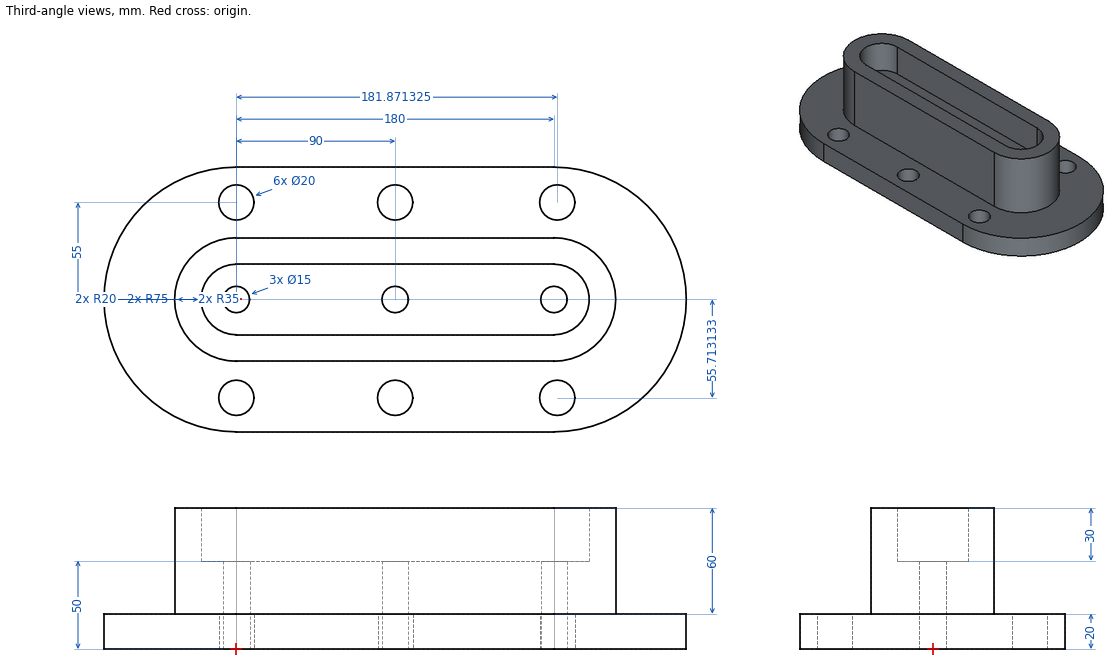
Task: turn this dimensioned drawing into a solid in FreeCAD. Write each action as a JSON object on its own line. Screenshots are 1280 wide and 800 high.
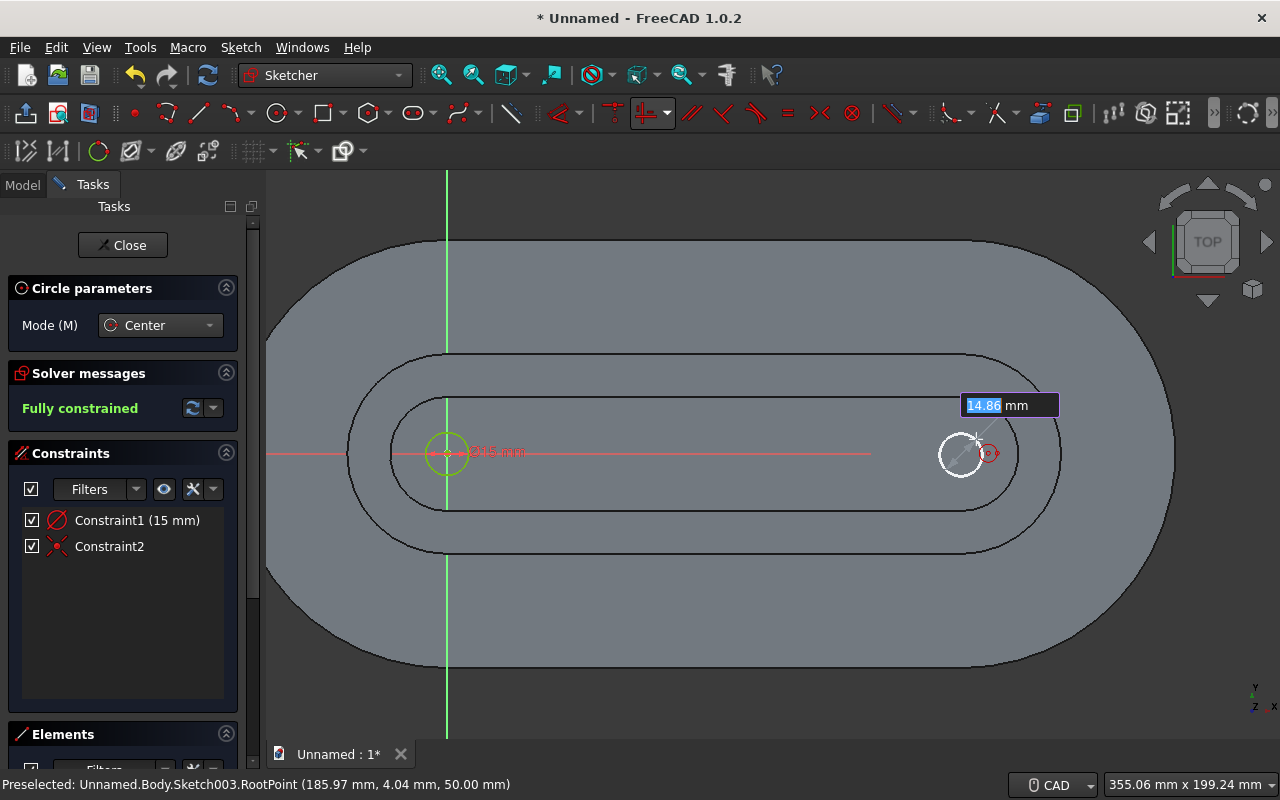
{"action": "type", "text": "15"}
{"action": "key", "text": "Return"}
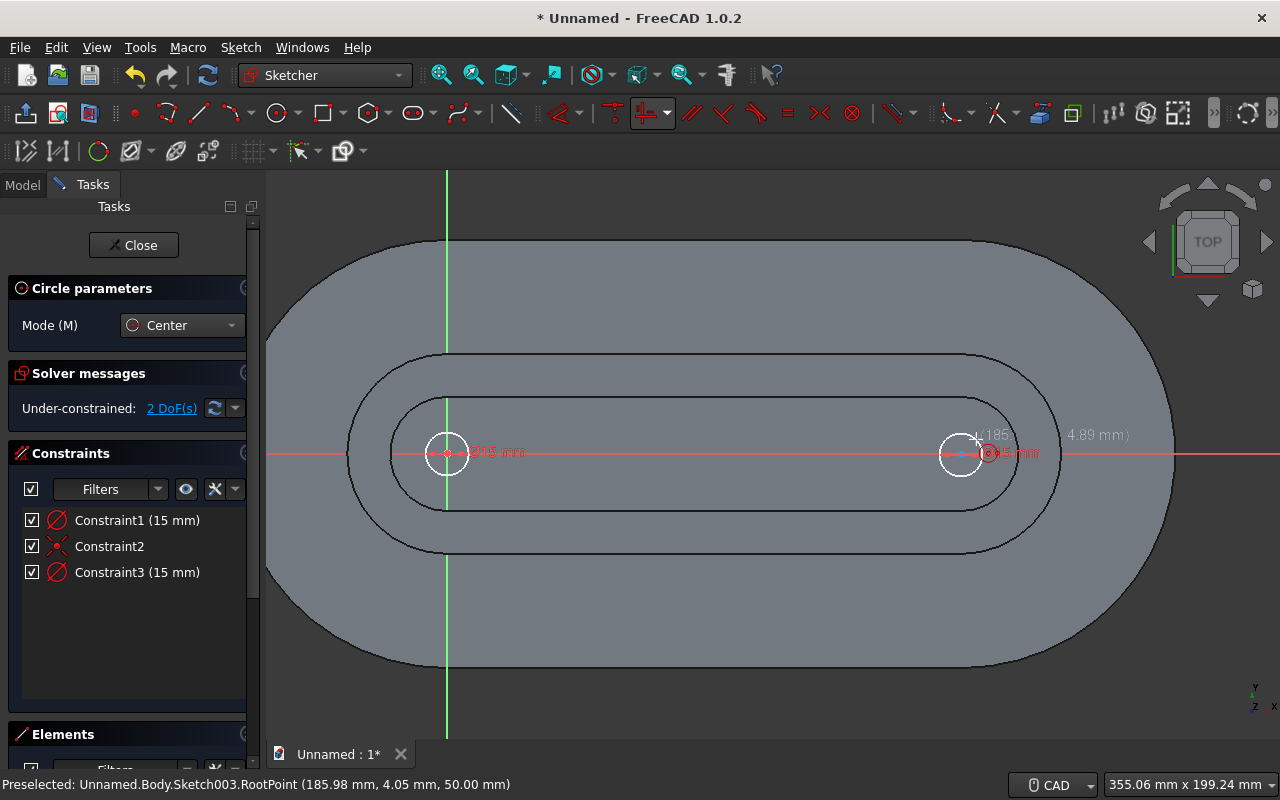
{"action": "left_click", "coordinate": [704, 454]}
{"action": "mouse_move", "coordinate": [719, 439]}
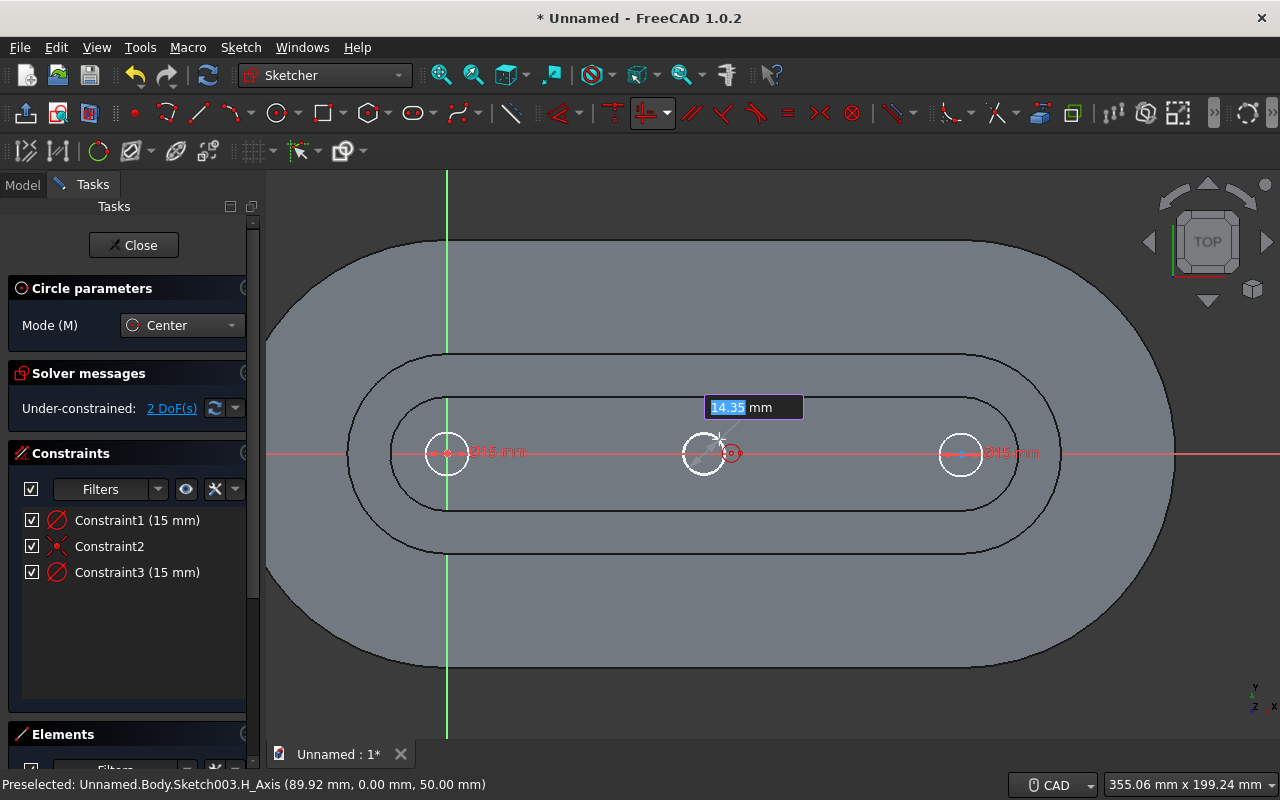
{"action": "type", "text": "15"}
{"action": "key", "text": "Return"}
{"action": "key", "text": "Escape"}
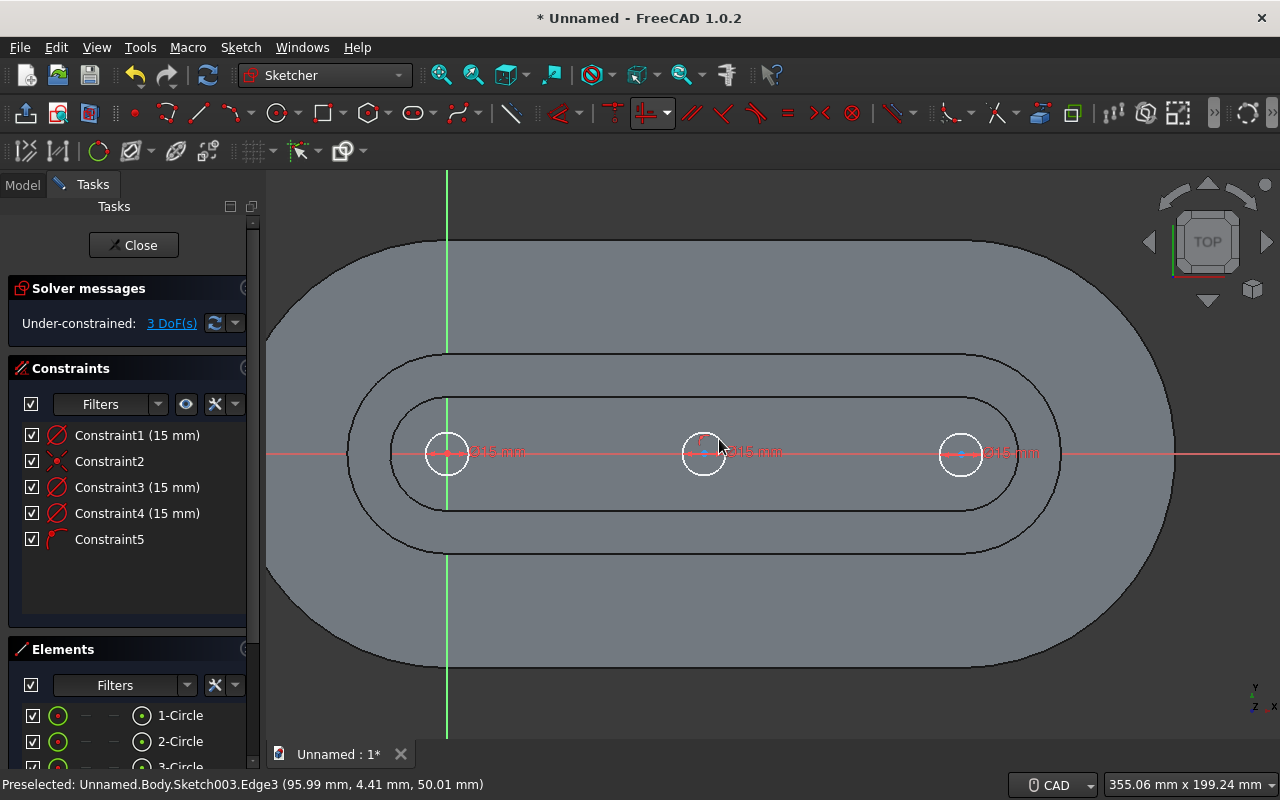
{"action": "left_click", "coordinate": [961, 455]}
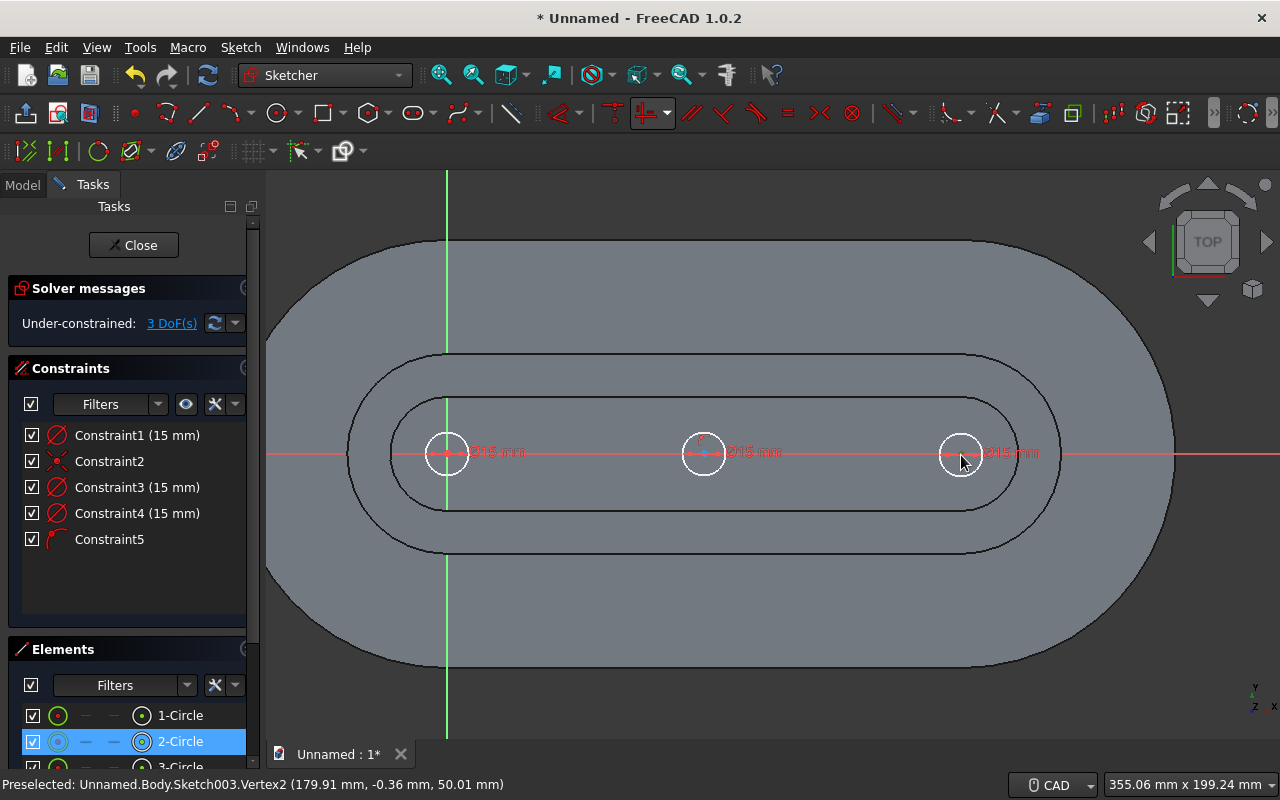
{"action": "left_click", "coordinate": [353, 454]}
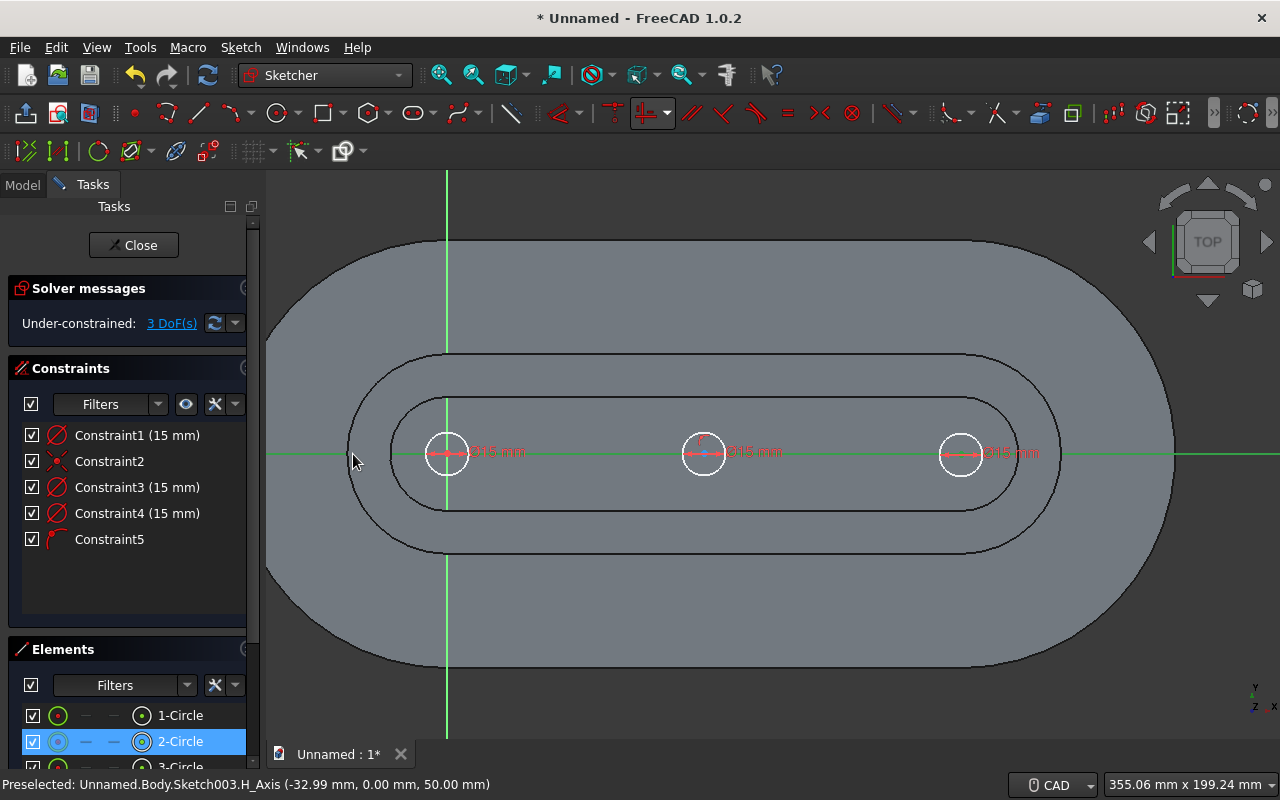
{"action": "key", "text": "c"}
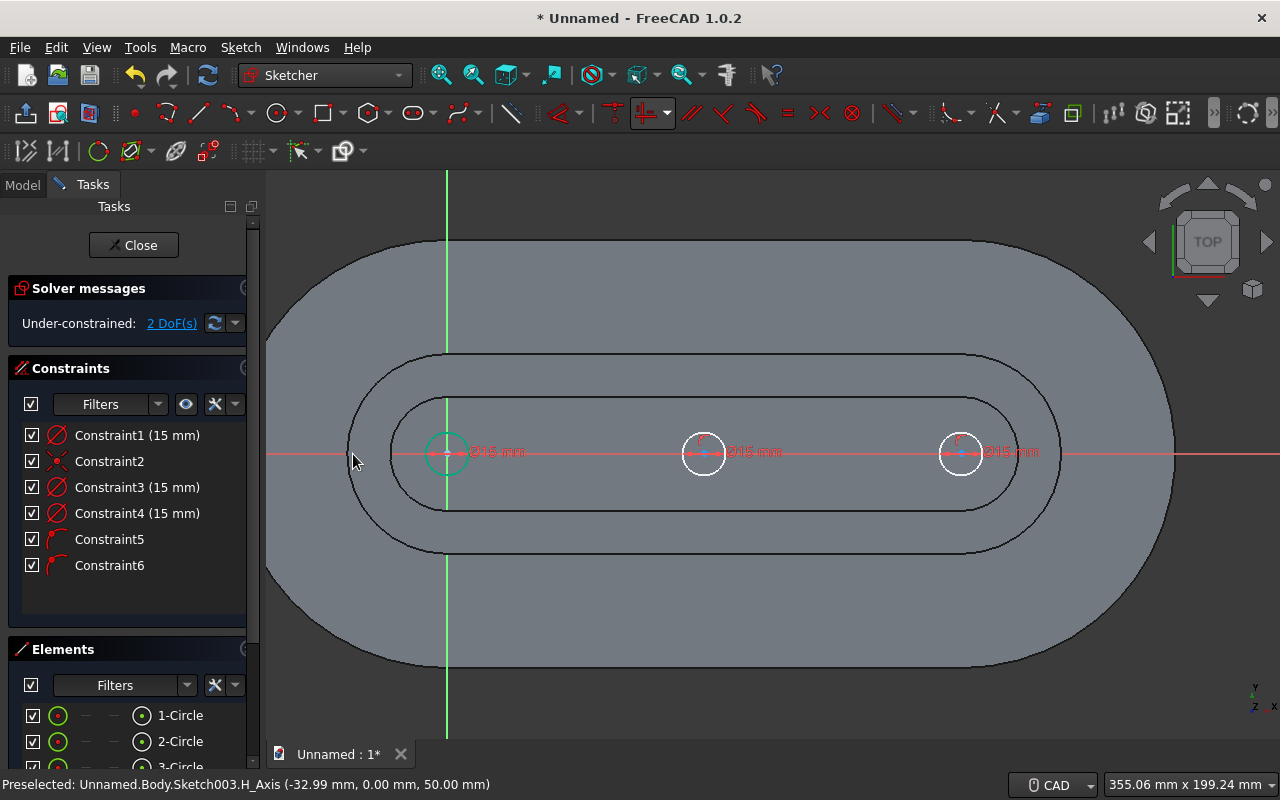
{"action": "key", "text": "d"}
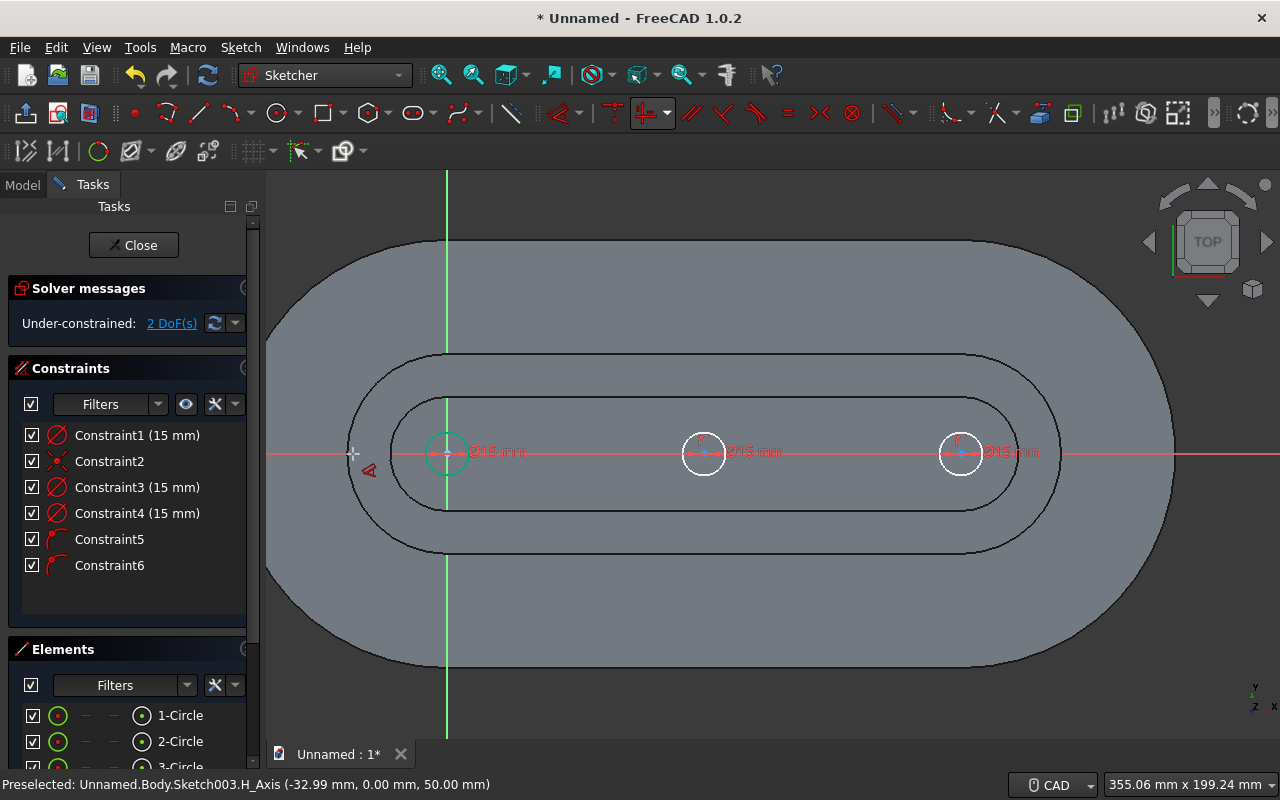
{"action": "left_click", "coordinate": [704, 454]}
{"action": "left_click", "coordinate": [576, 488]}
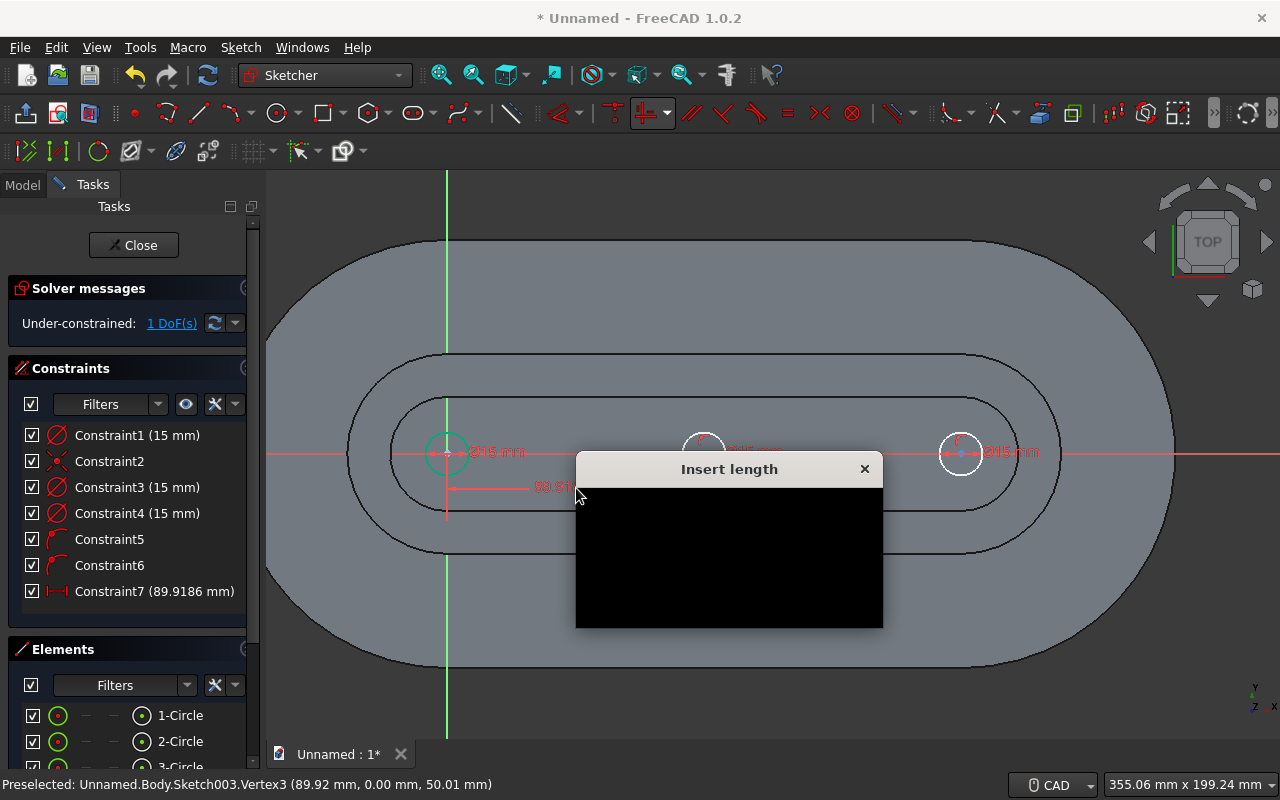
{"action": "type", "text": "90"}
{"action": "key", "text": "Return"}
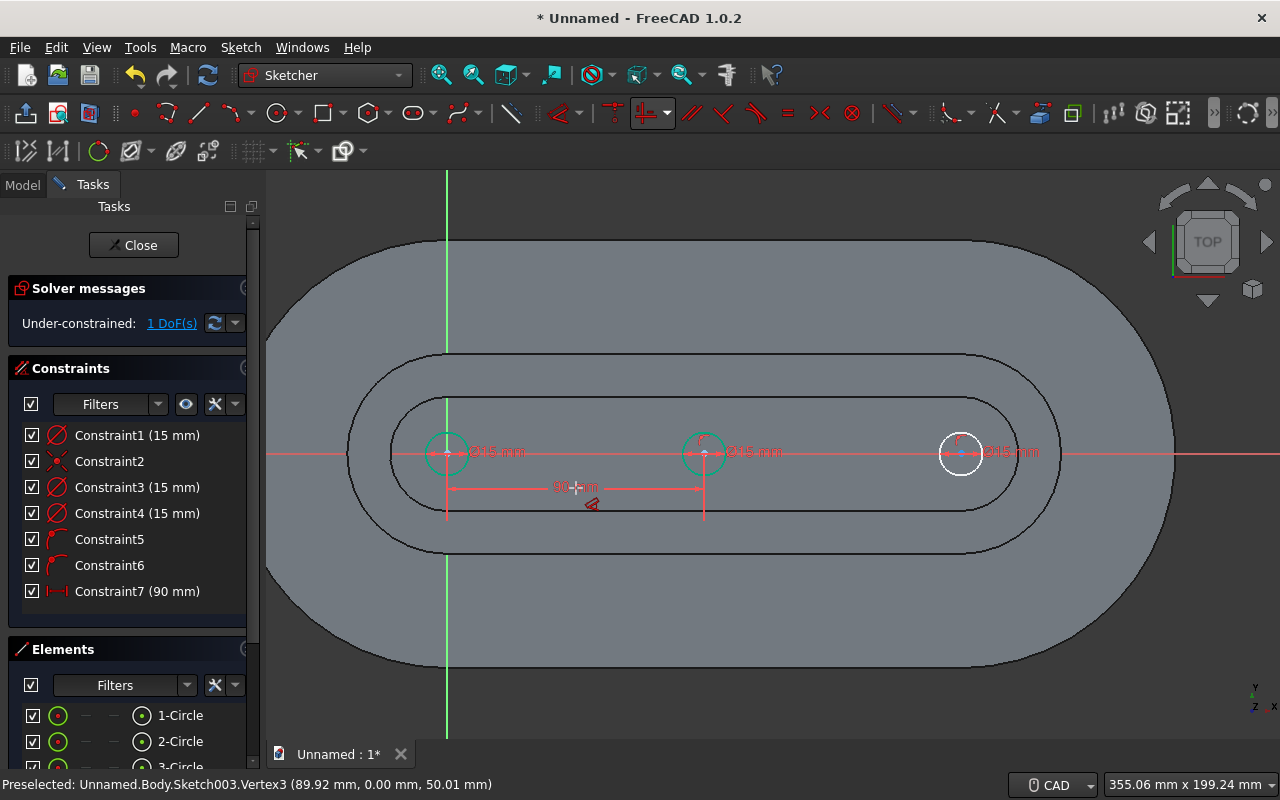
{"action": "left_click", "coordinate": [961, 454]}
{"action": "left_click", "coordinate": [822, 488]}